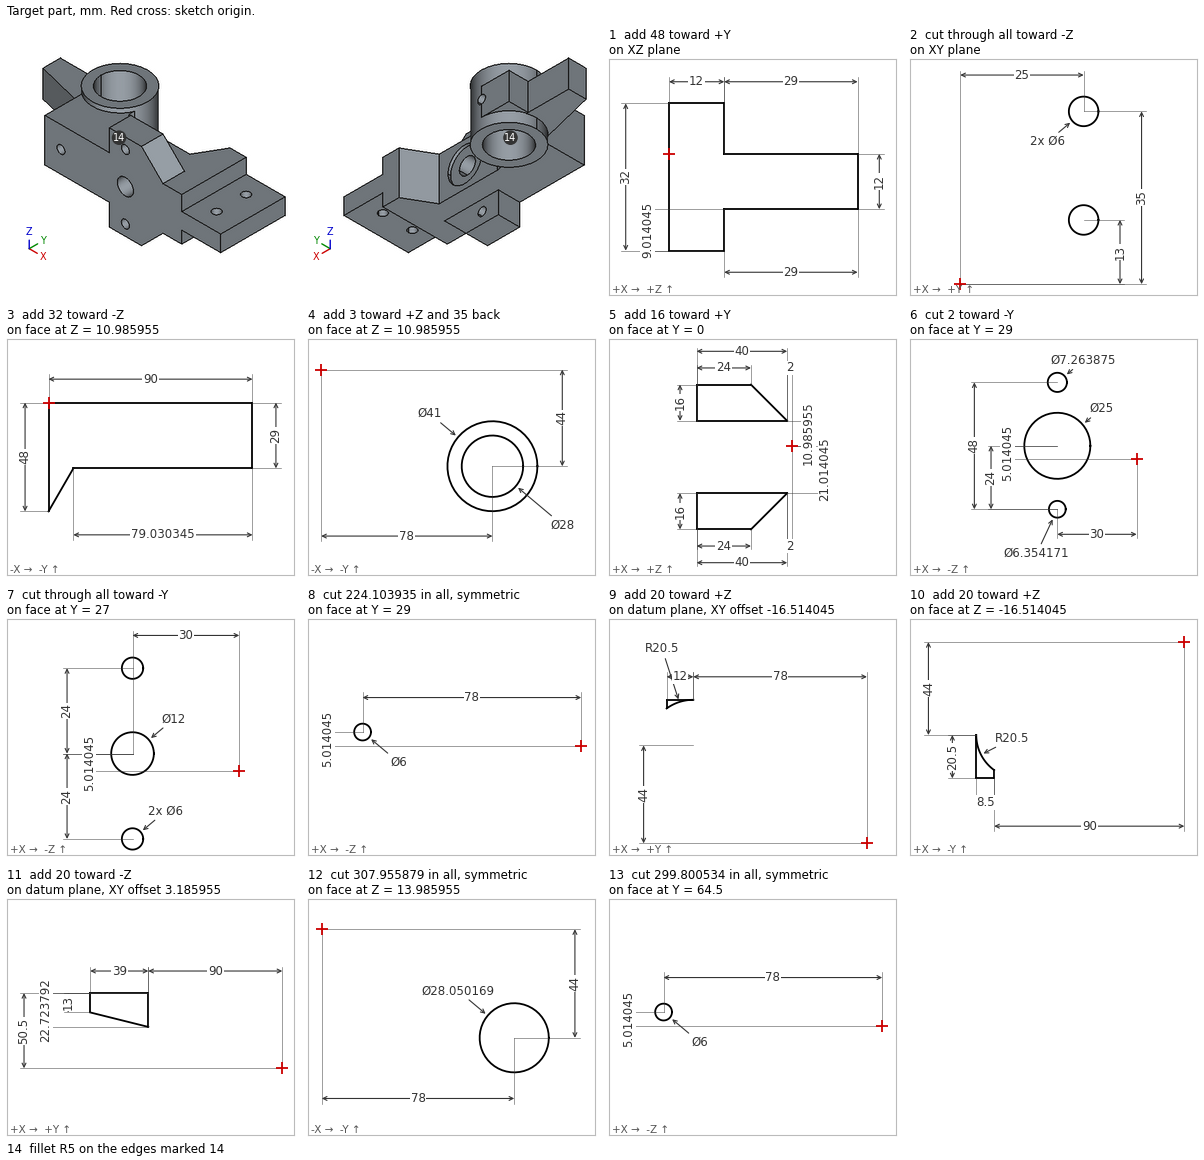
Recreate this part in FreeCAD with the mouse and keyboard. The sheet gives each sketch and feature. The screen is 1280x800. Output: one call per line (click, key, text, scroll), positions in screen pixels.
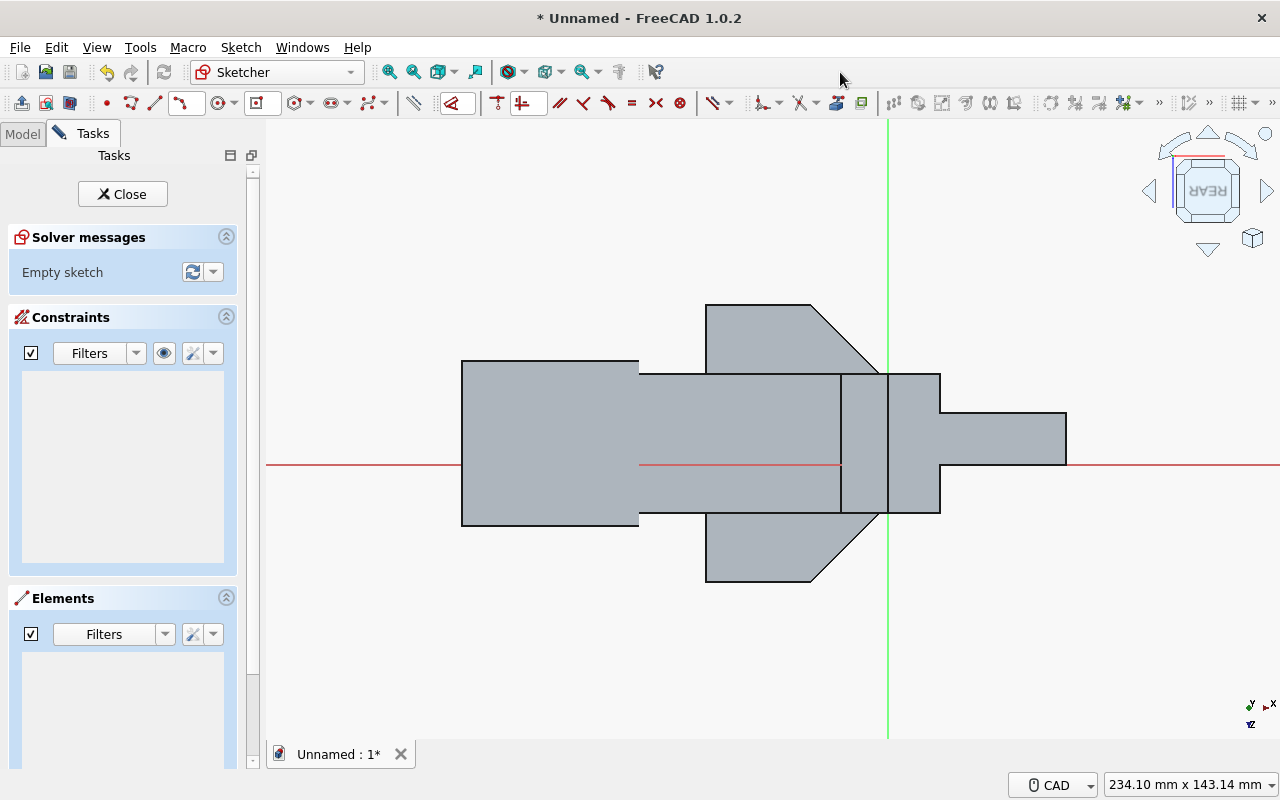
key(q)
key(s)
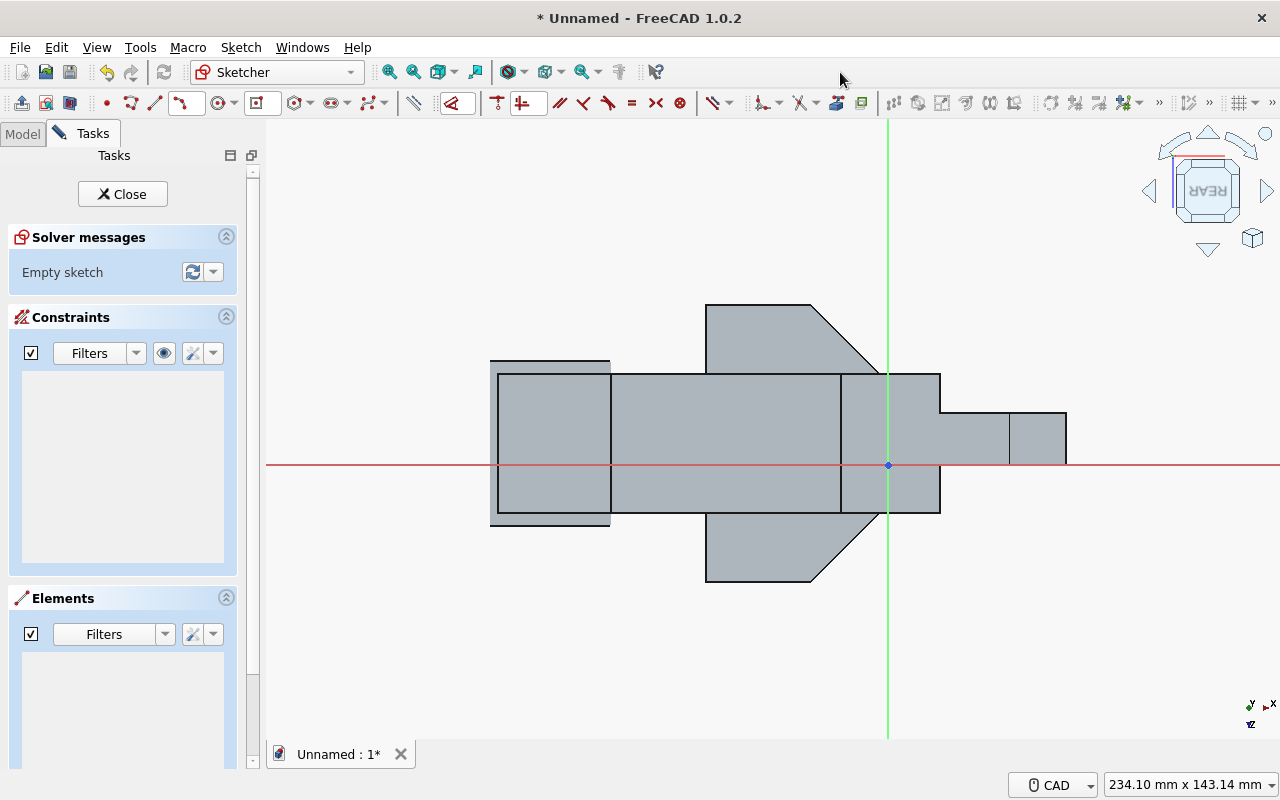
scroll(908, 459, up, 3)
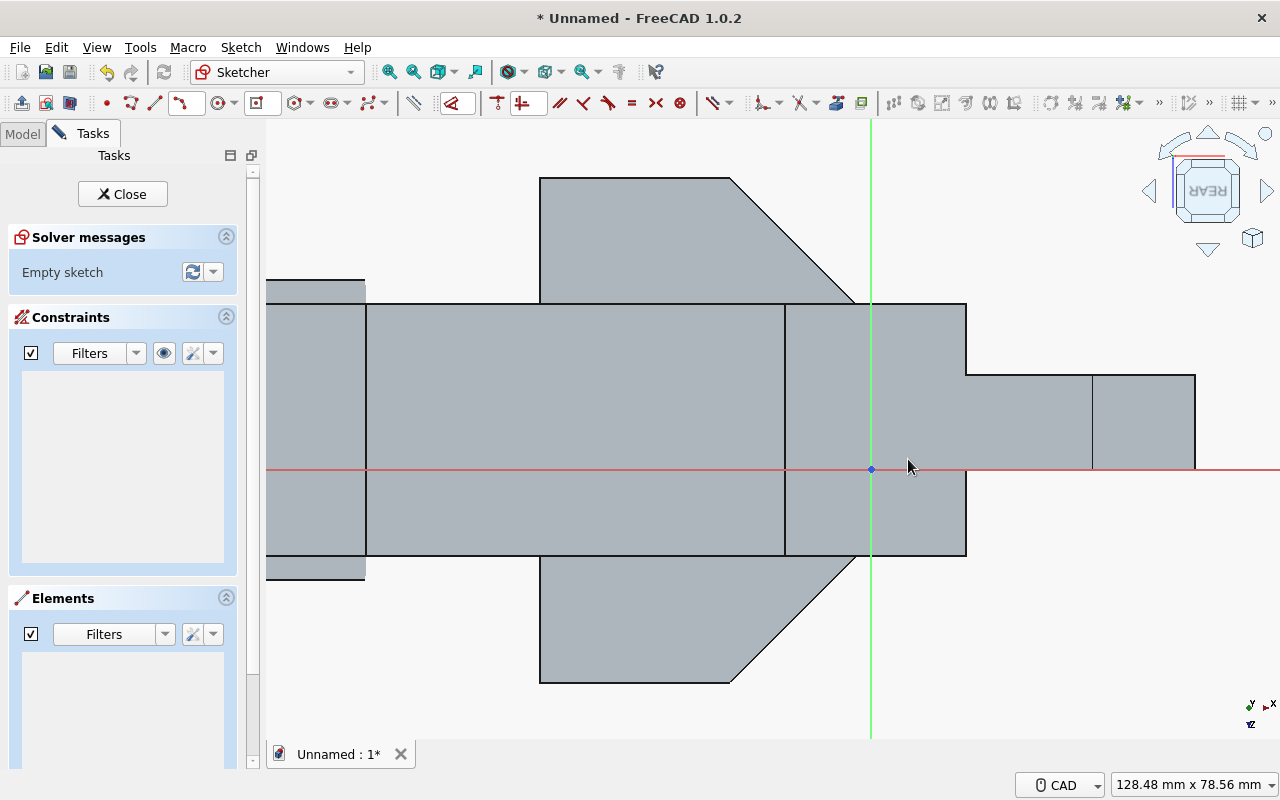
key(g)
key(c)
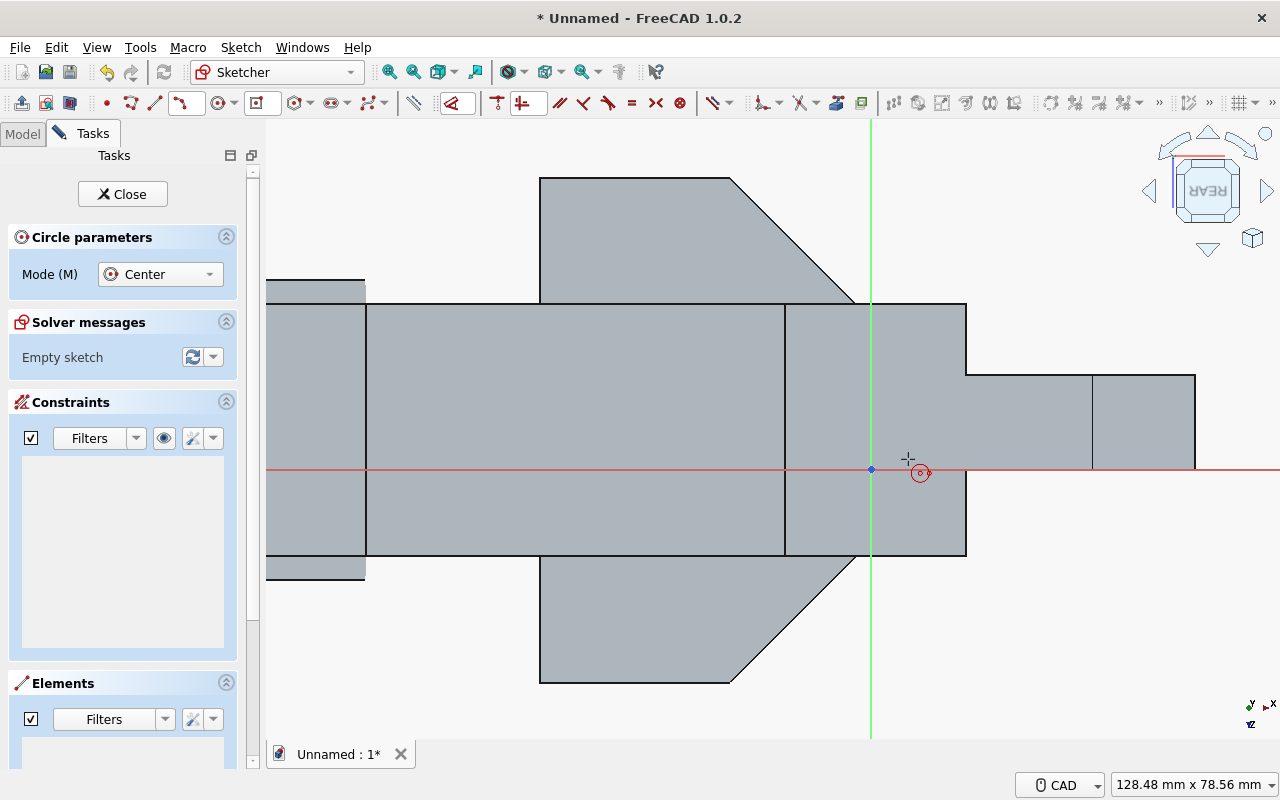
click(635, 620)
move(652, 602)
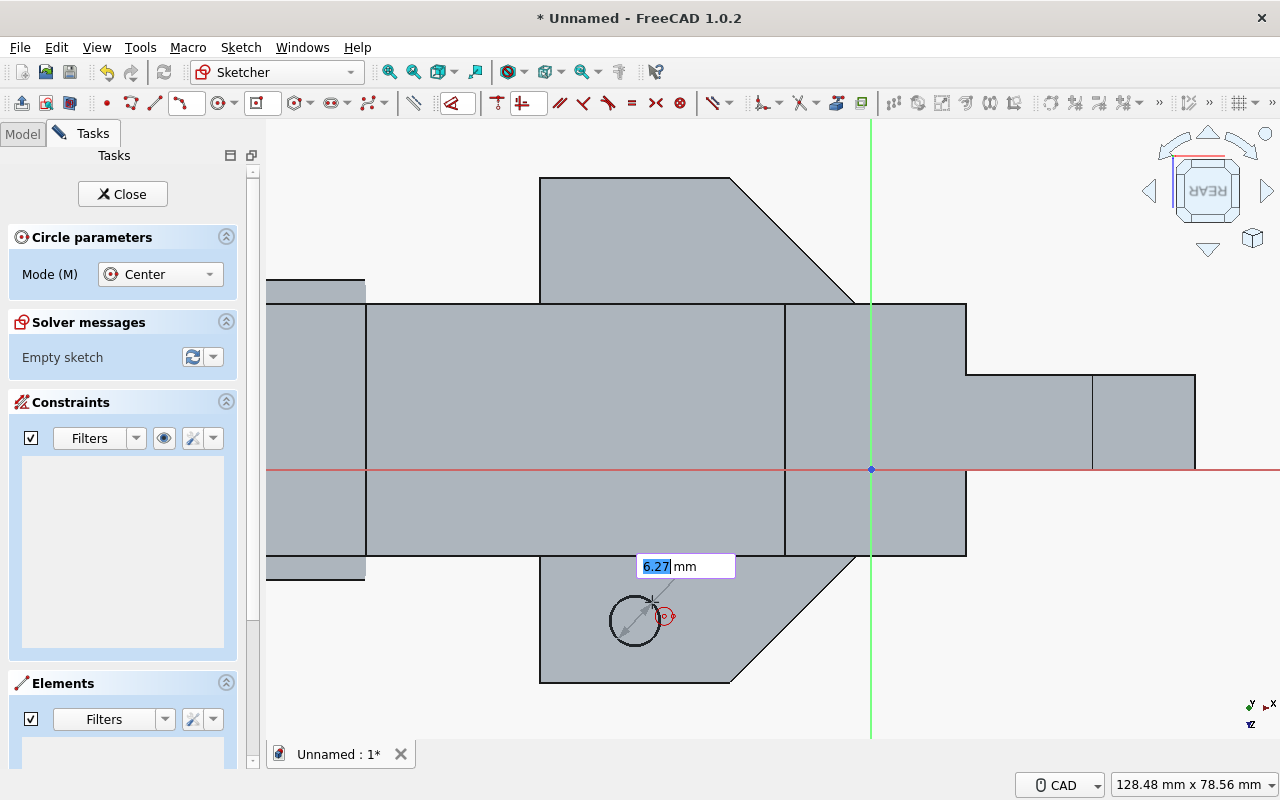
text(6.354171)
key(Return)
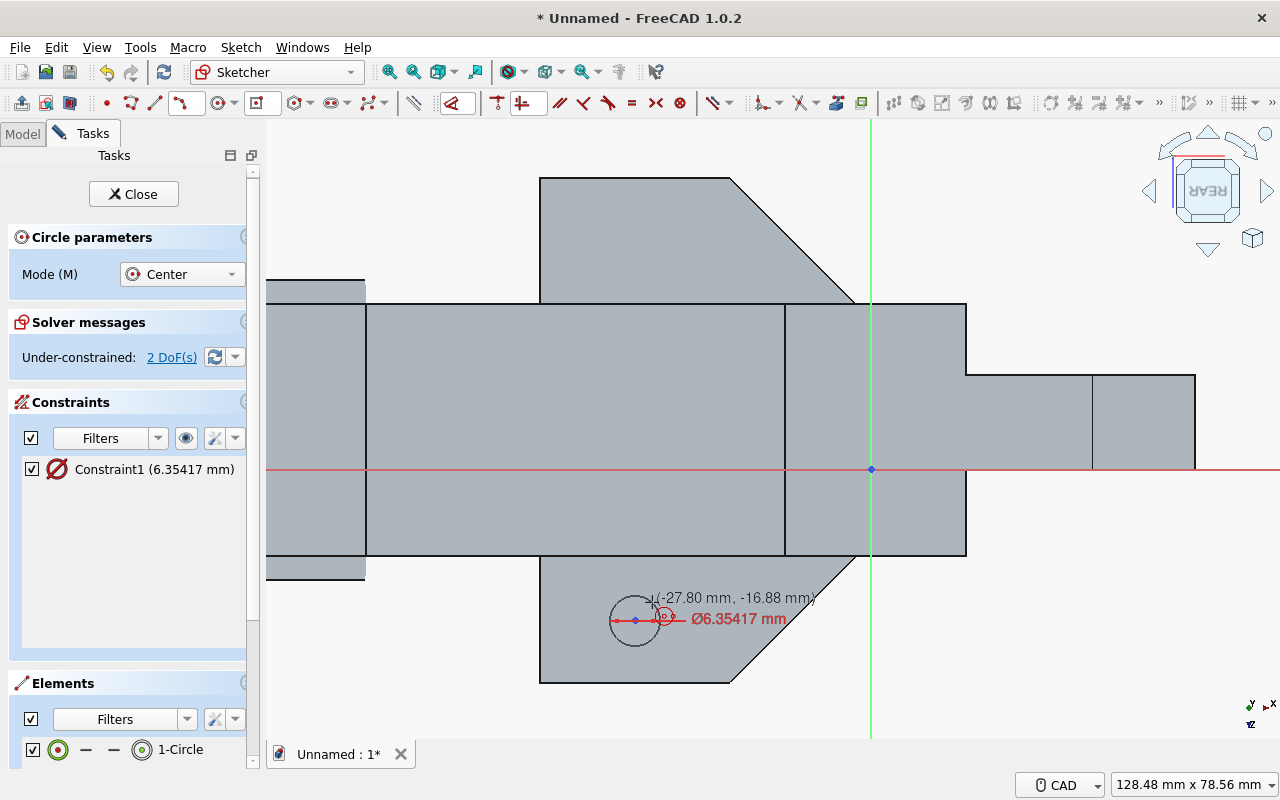
click(635, 241)
move(655, 221)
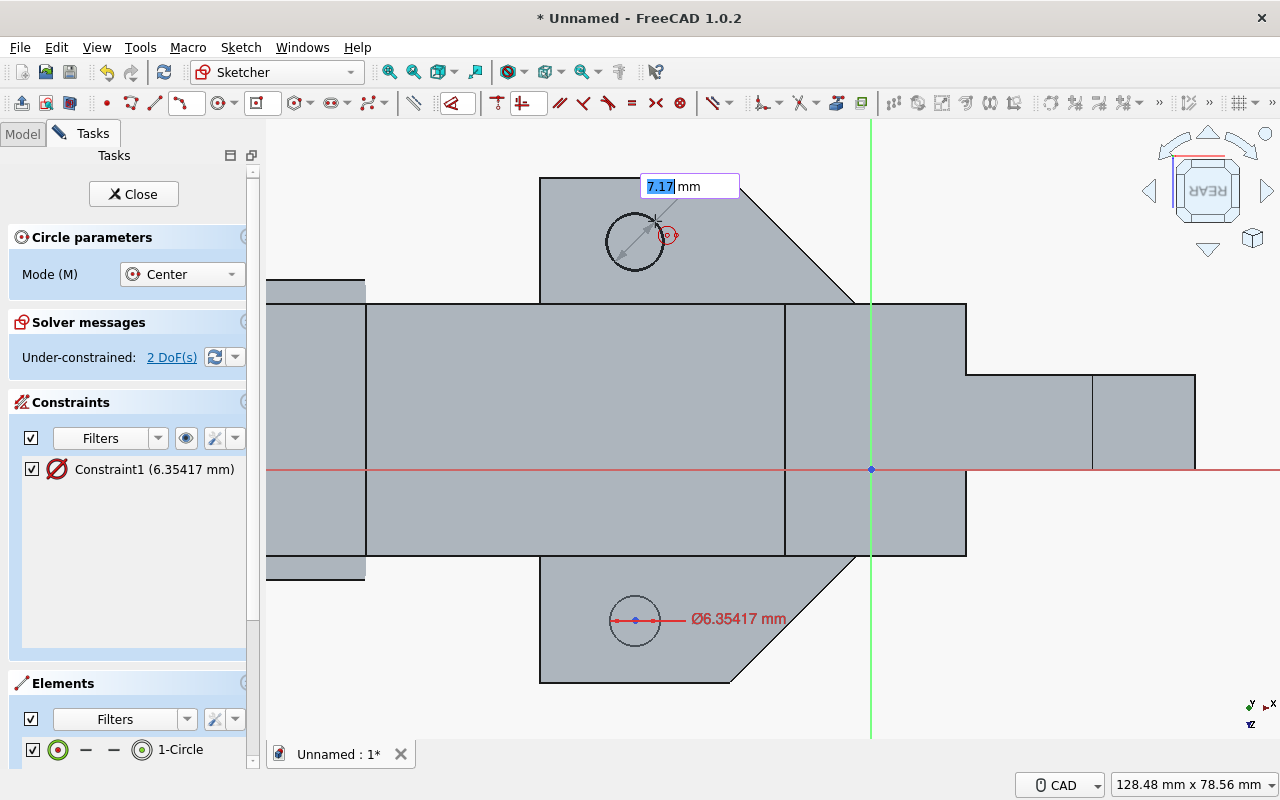
text(7.263875)
key(Return)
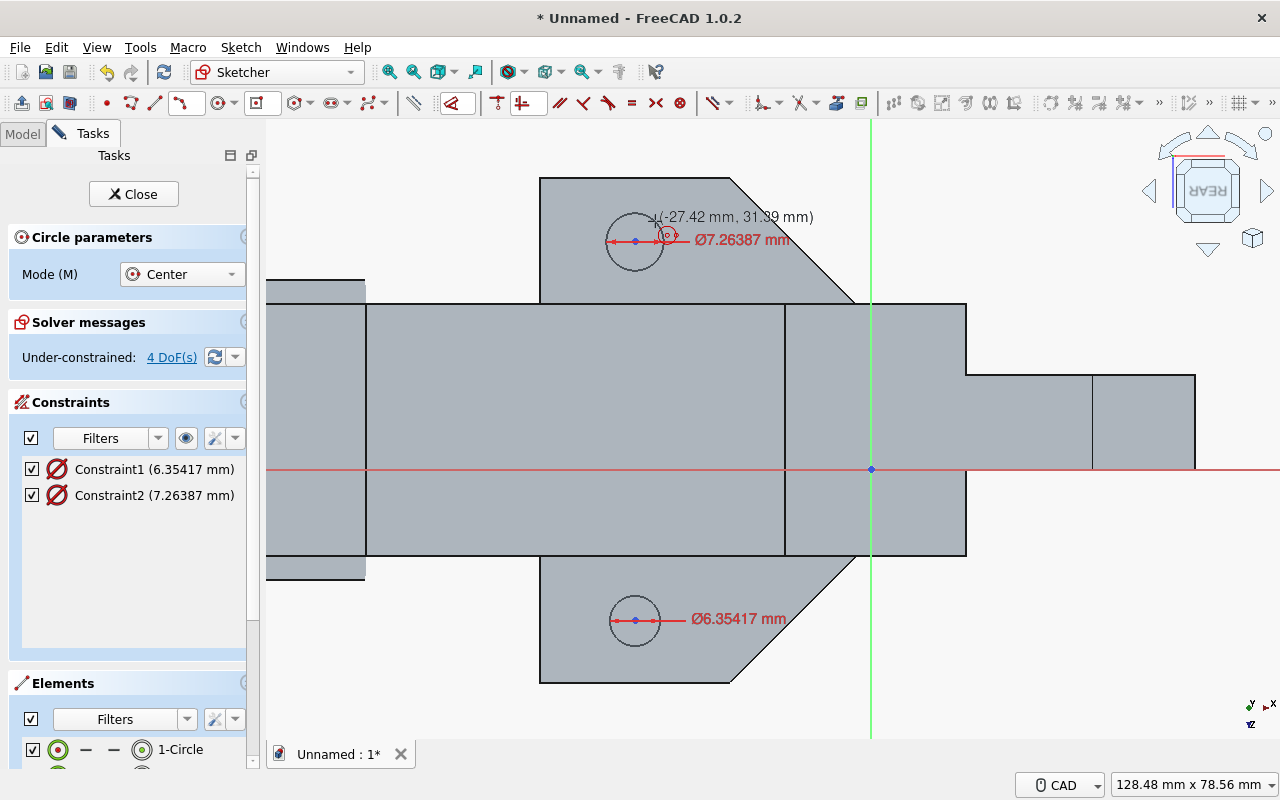
click(635, 430)
move(704, 360)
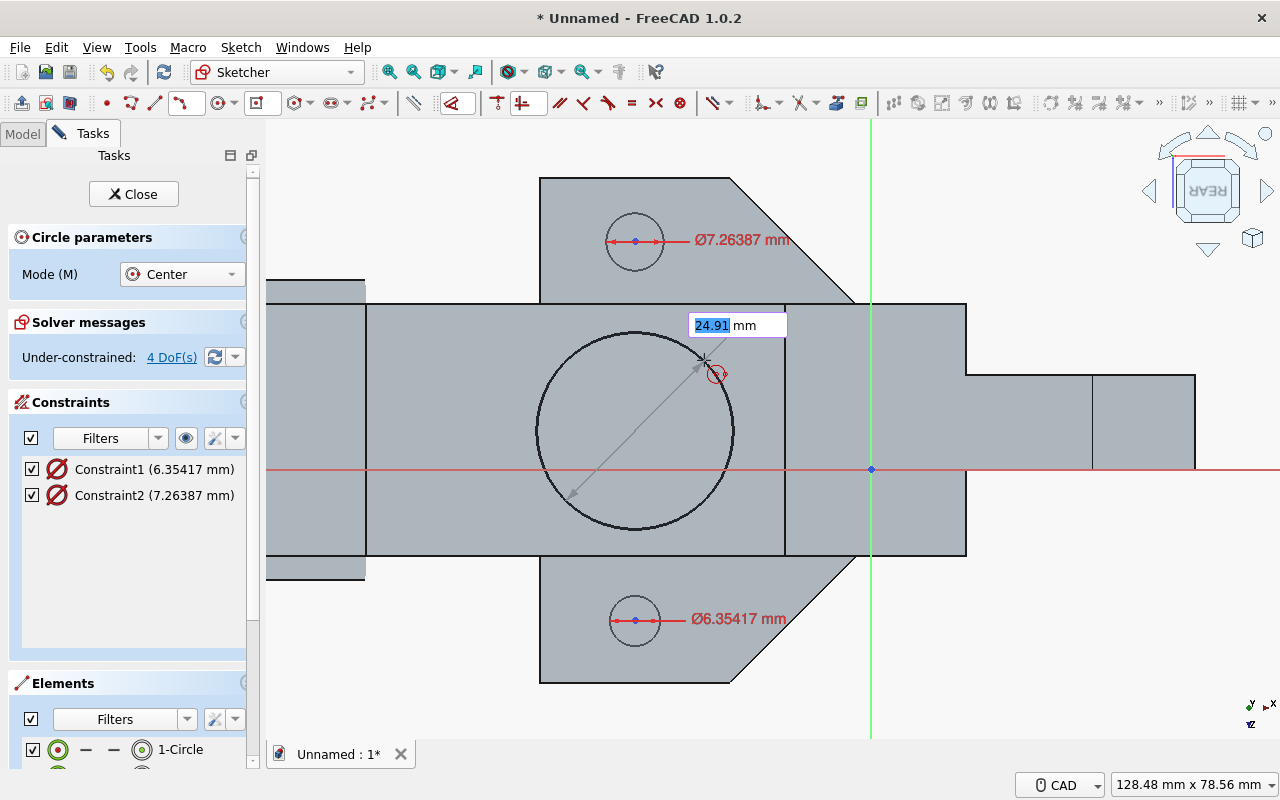
text(25)
key(Return)
key(Escape)